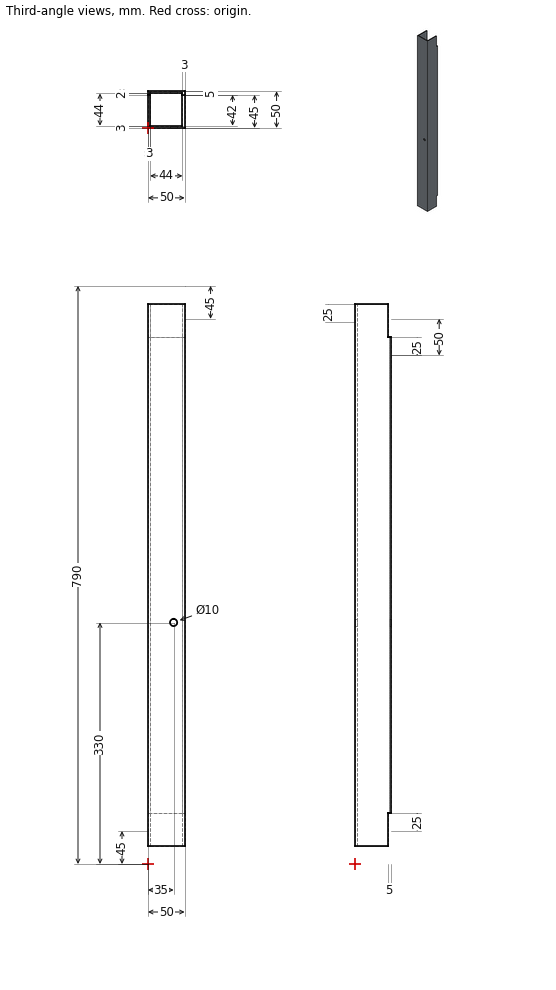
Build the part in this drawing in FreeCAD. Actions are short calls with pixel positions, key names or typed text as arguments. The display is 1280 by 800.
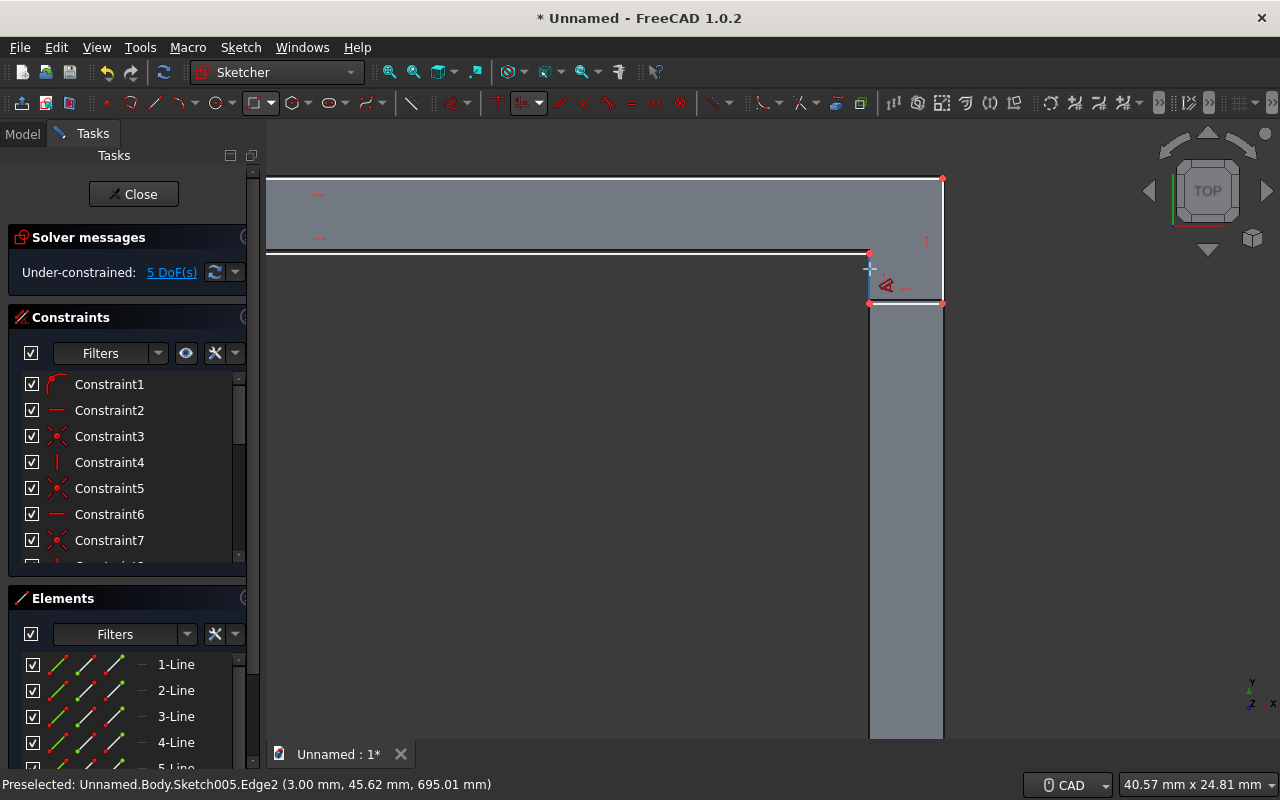
click(869, 269)
click(903, 279)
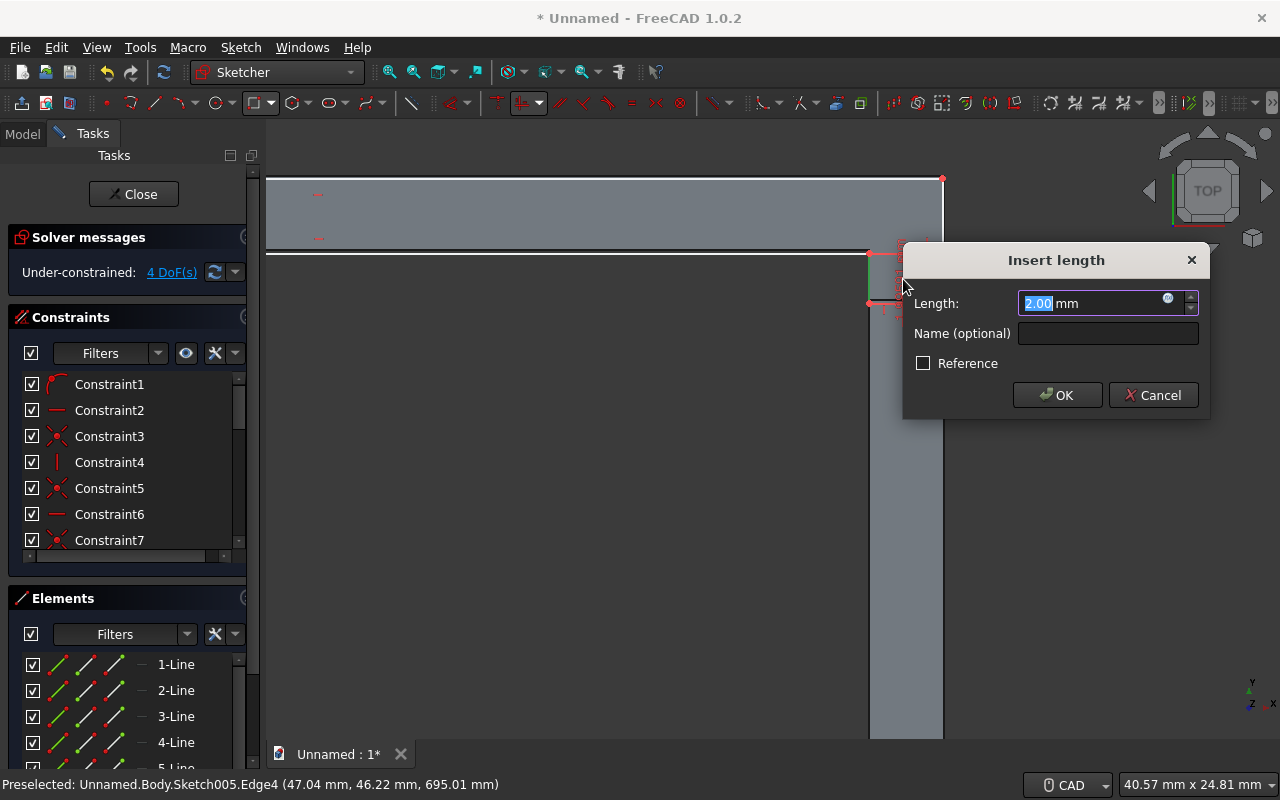
text(2)
key(Return)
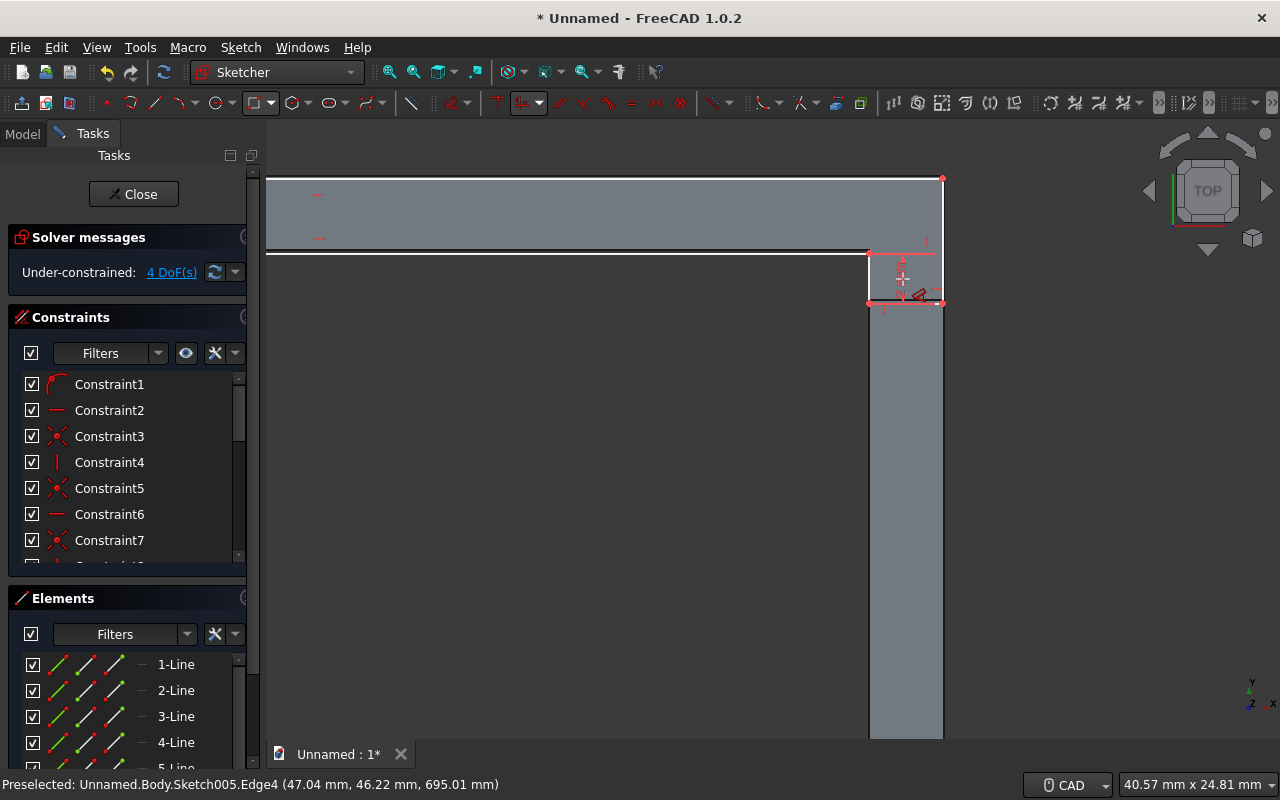
click(891, 304)
click(906, 338)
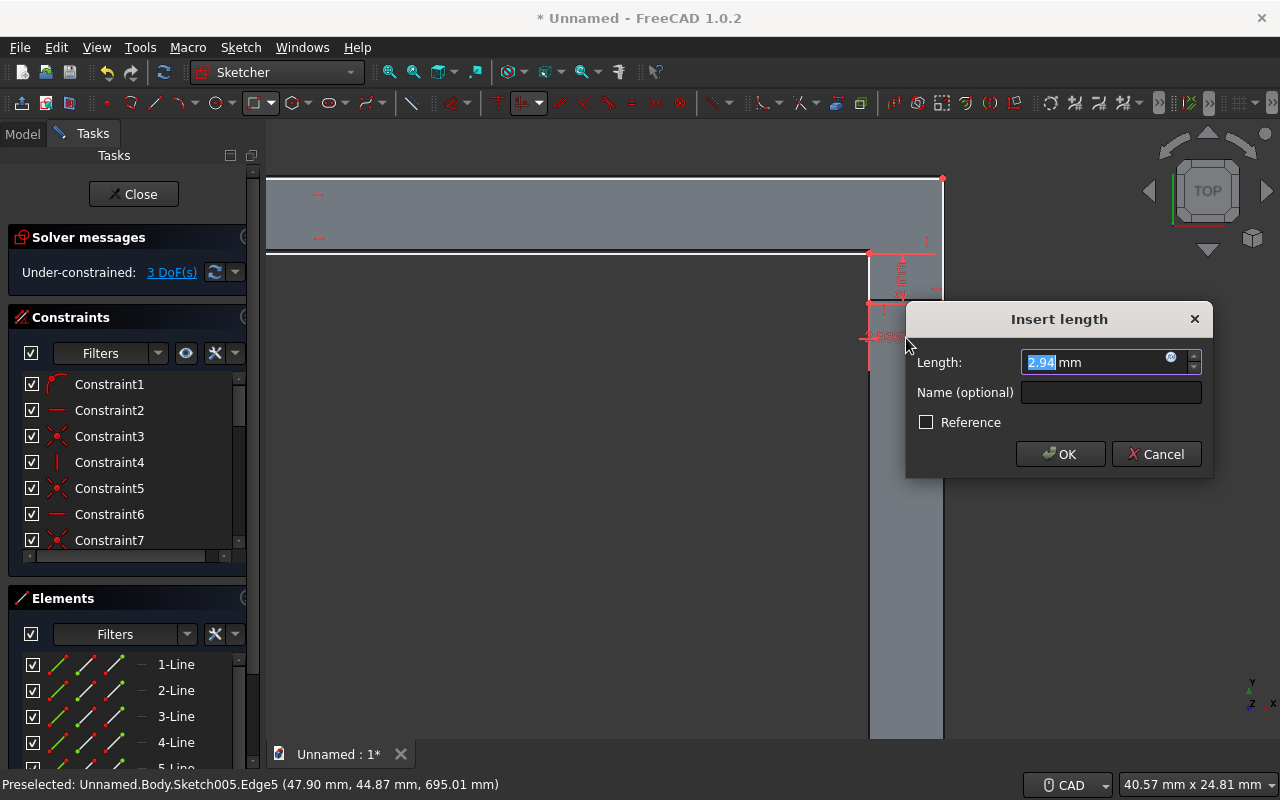
text(3)
key(Return)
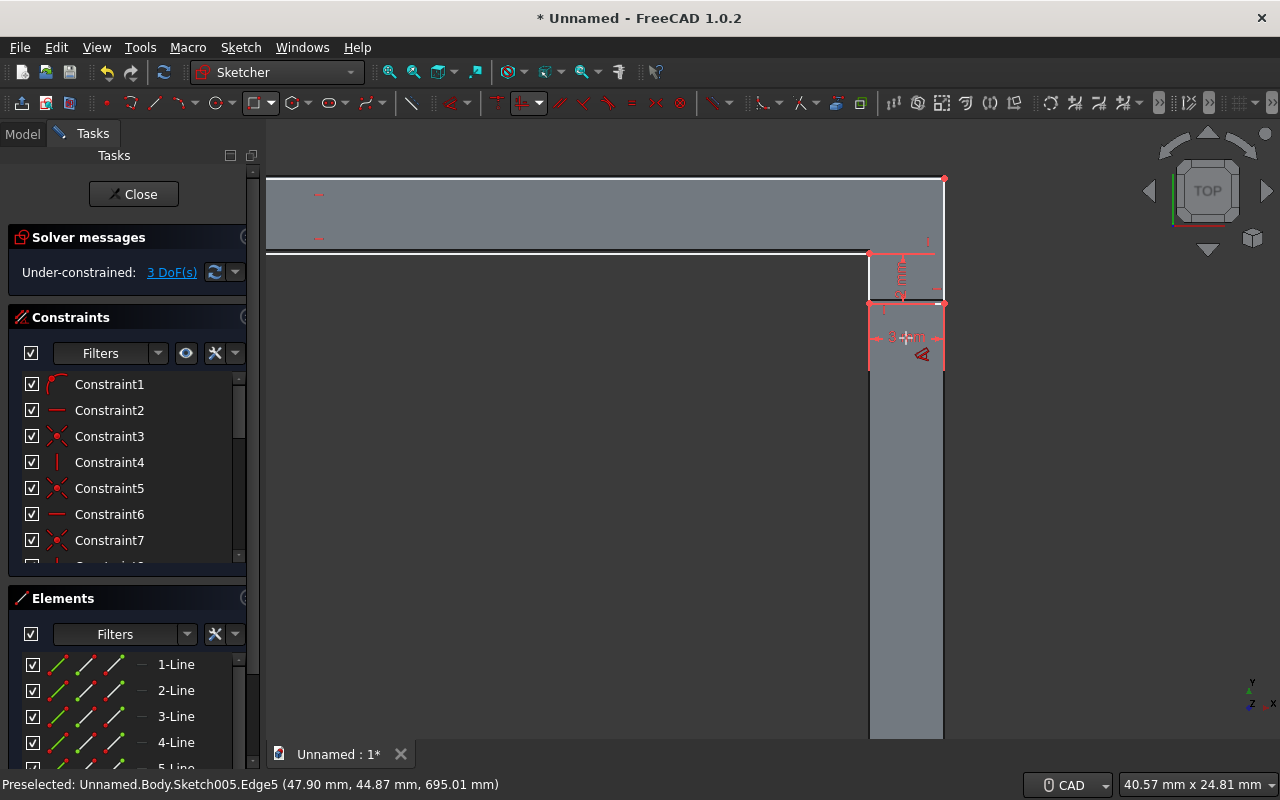
click(944, 266)
click(978, 241)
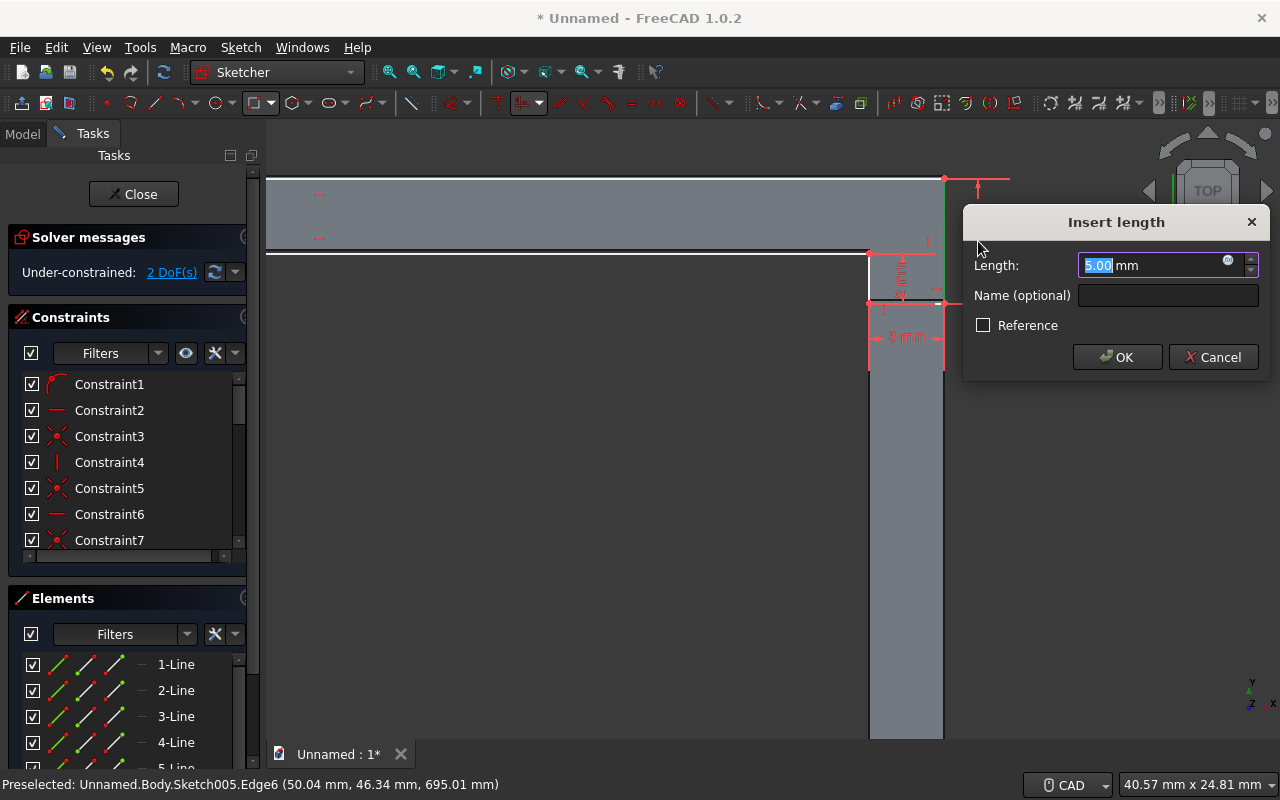
text(5)
key(Return)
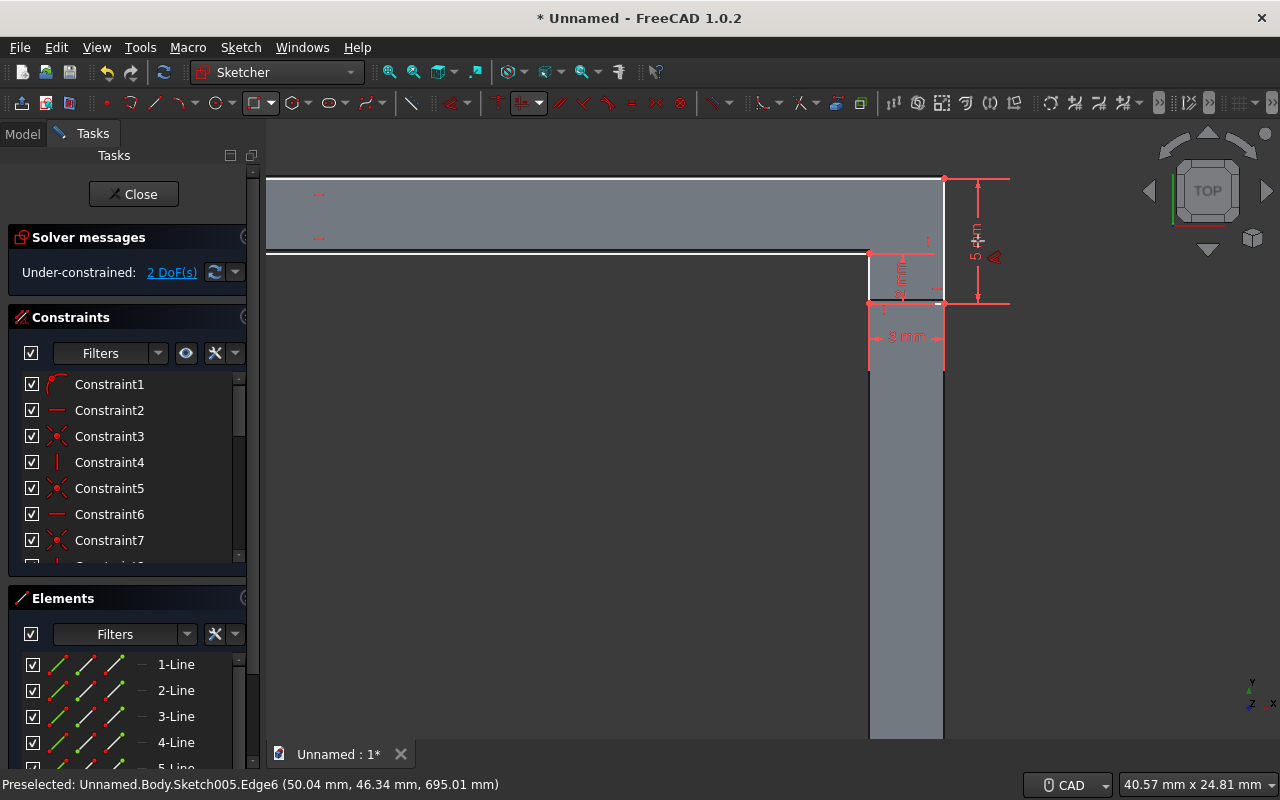
scroll(871, 269, down, 6)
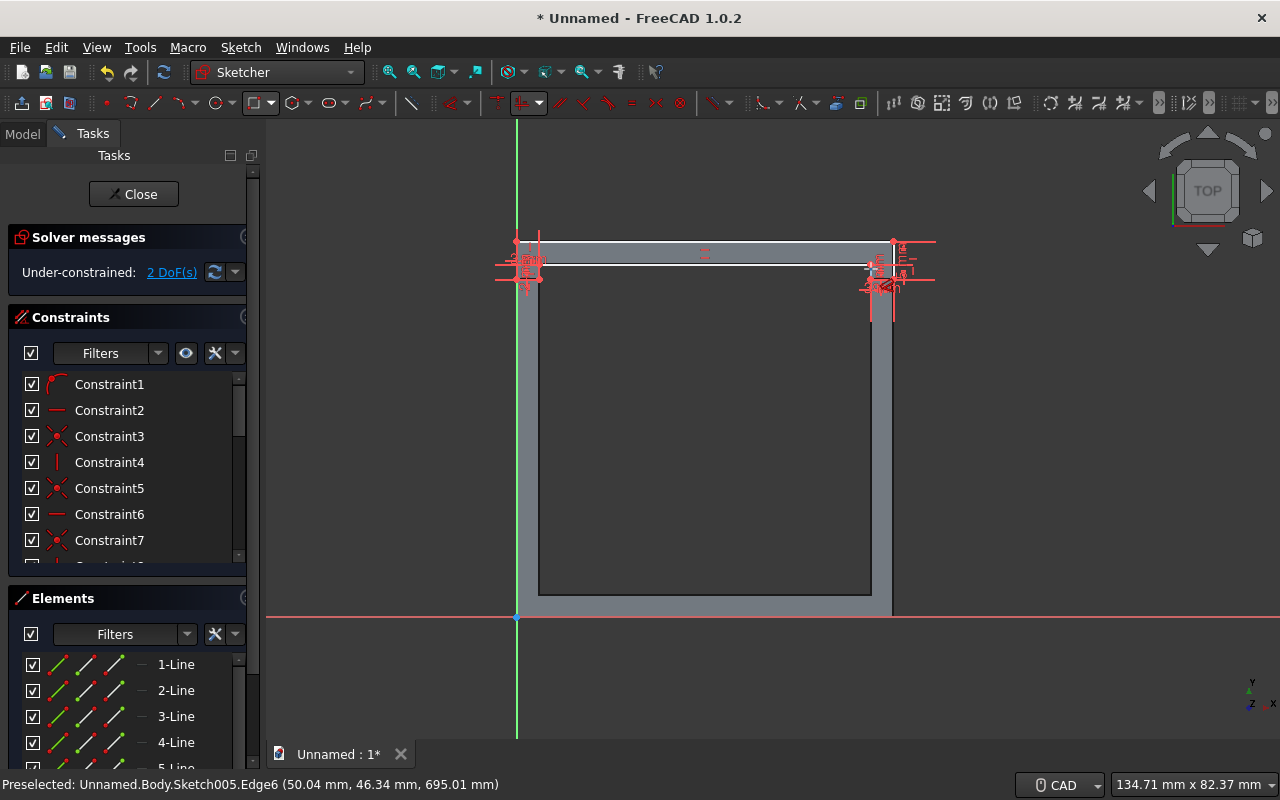
click(772, 265)
click(705, 299)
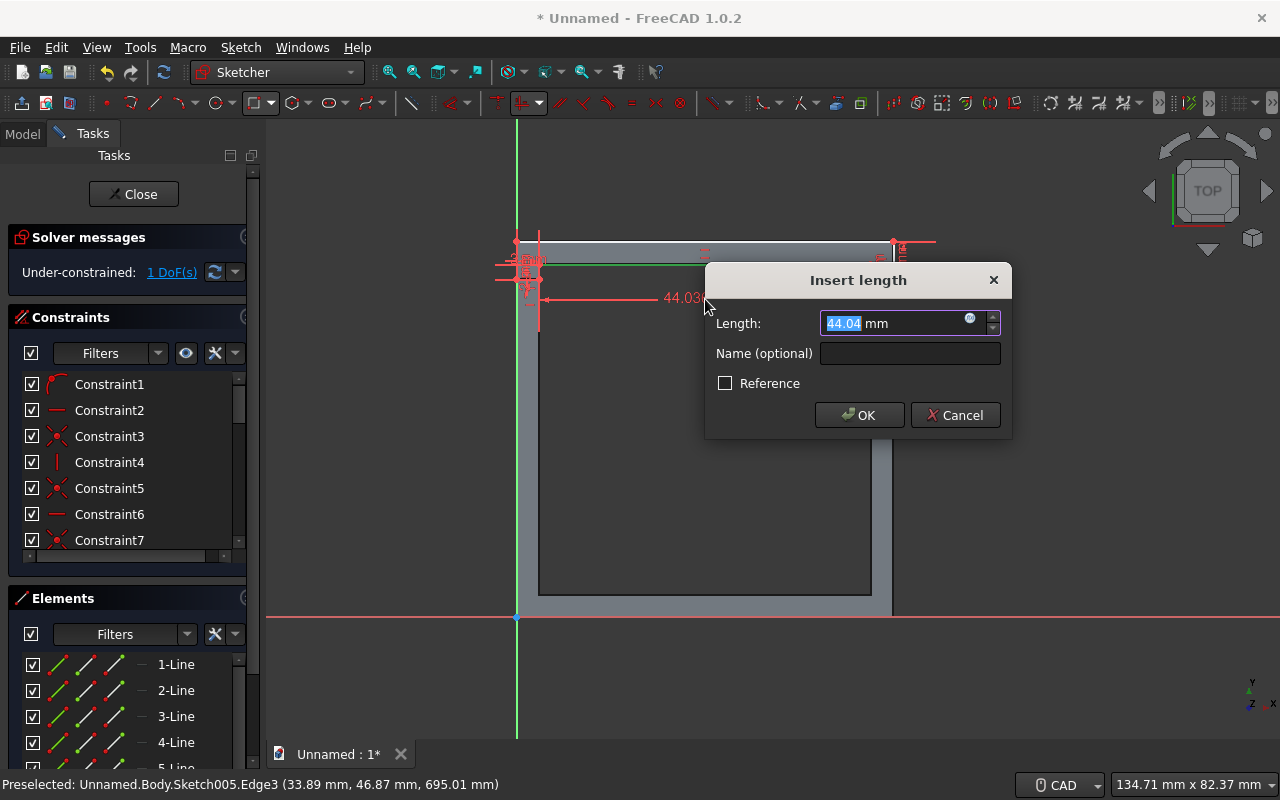
text(44)
key(Return)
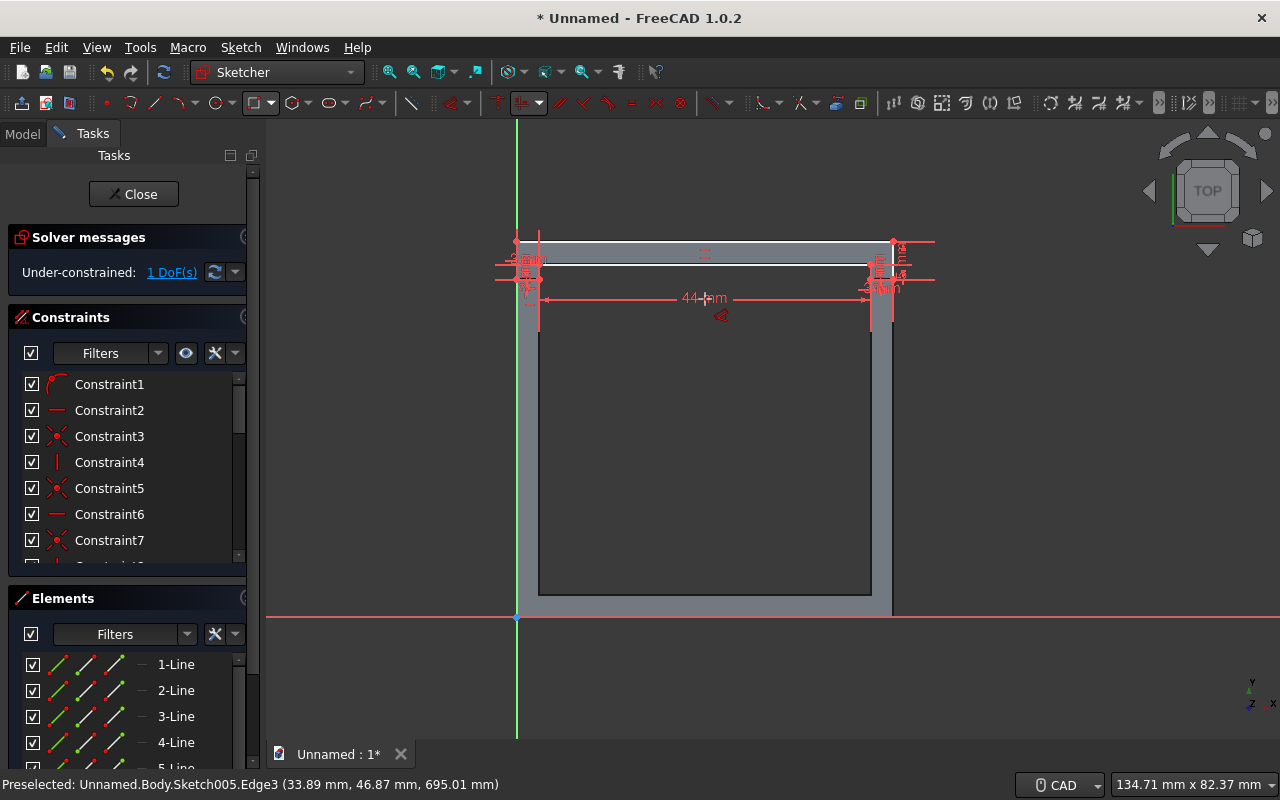
click(517, 280)
click(483, 448)